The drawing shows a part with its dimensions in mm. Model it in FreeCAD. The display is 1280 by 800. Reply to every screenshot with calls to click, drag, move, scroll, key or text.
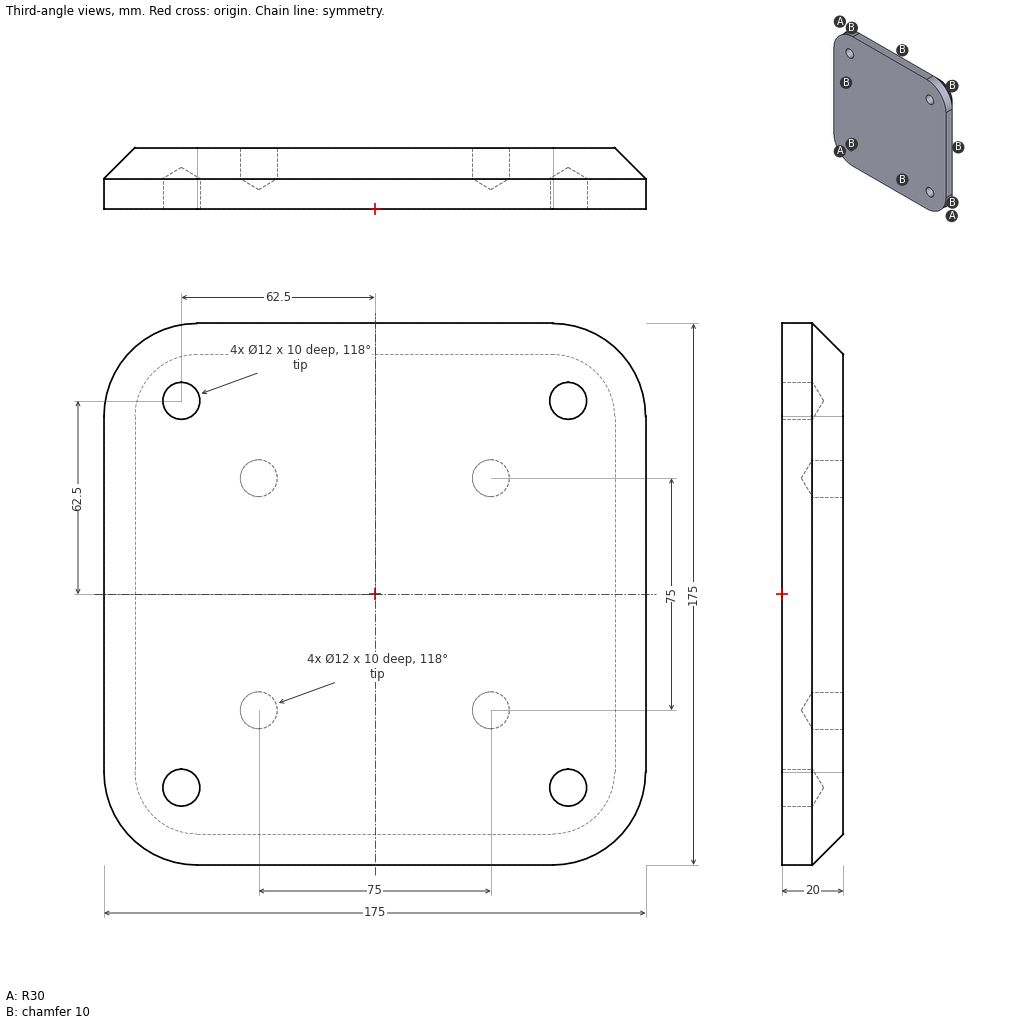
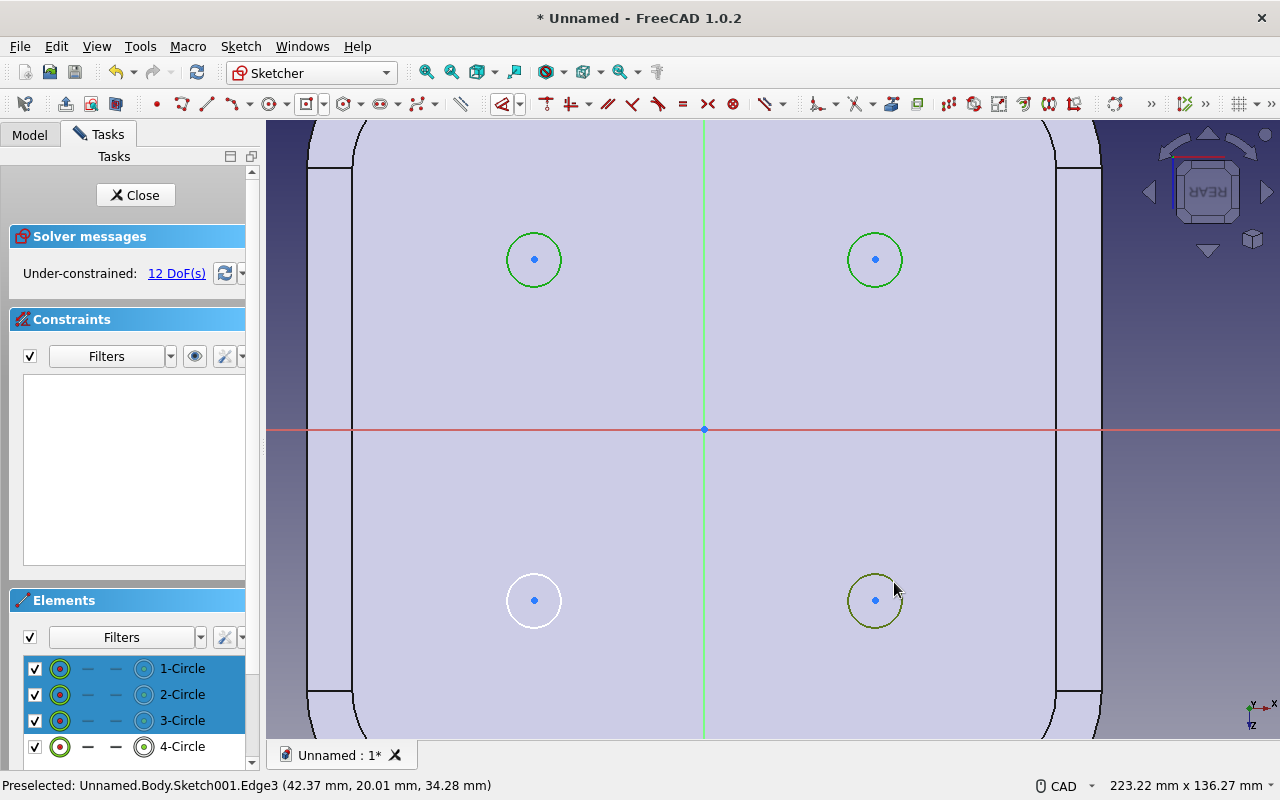
click(553, 582)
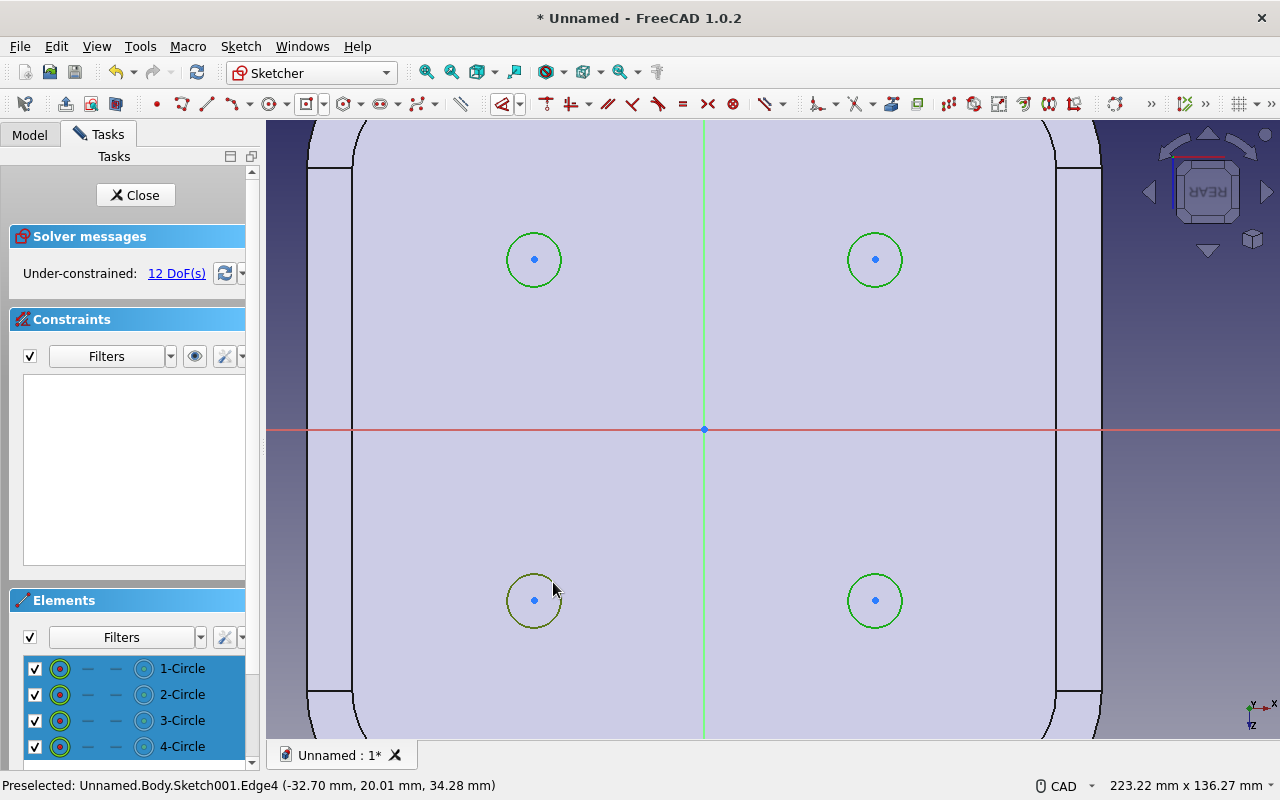
click(683, 104)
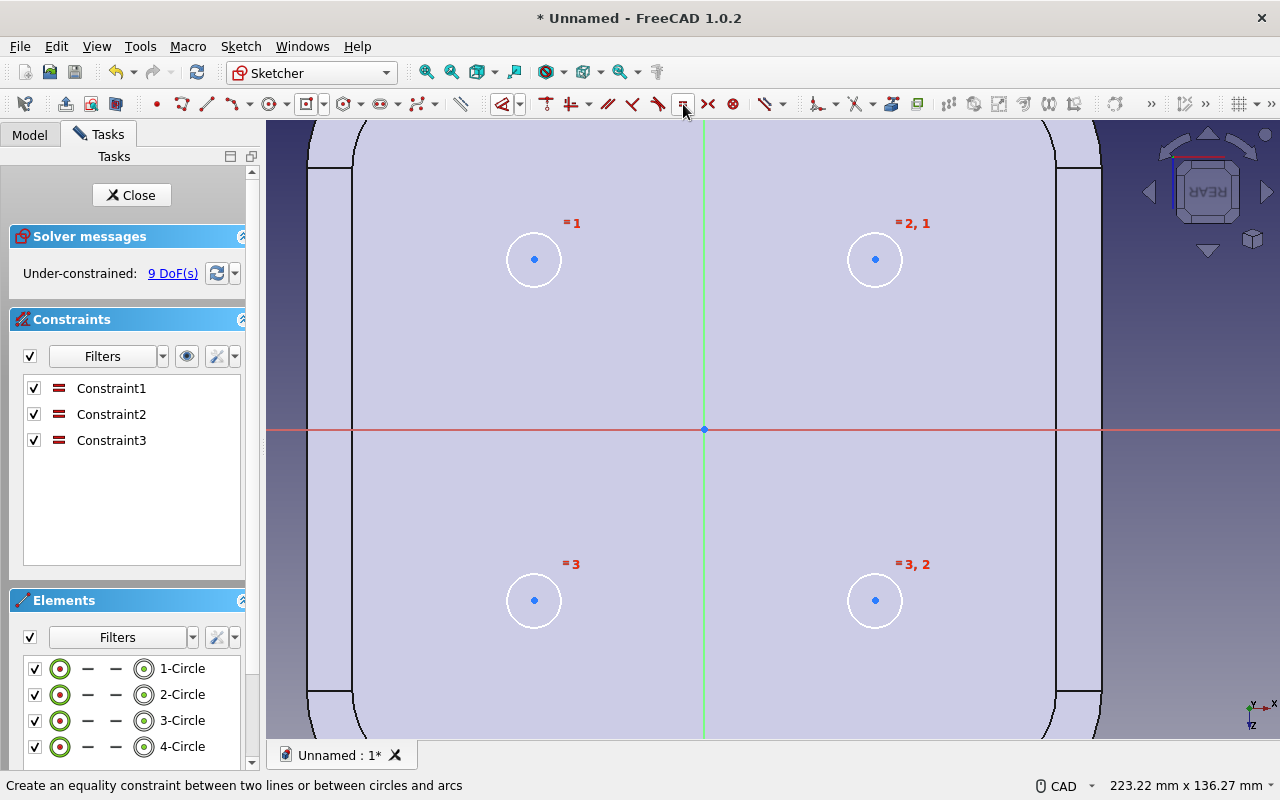
click(534, 260)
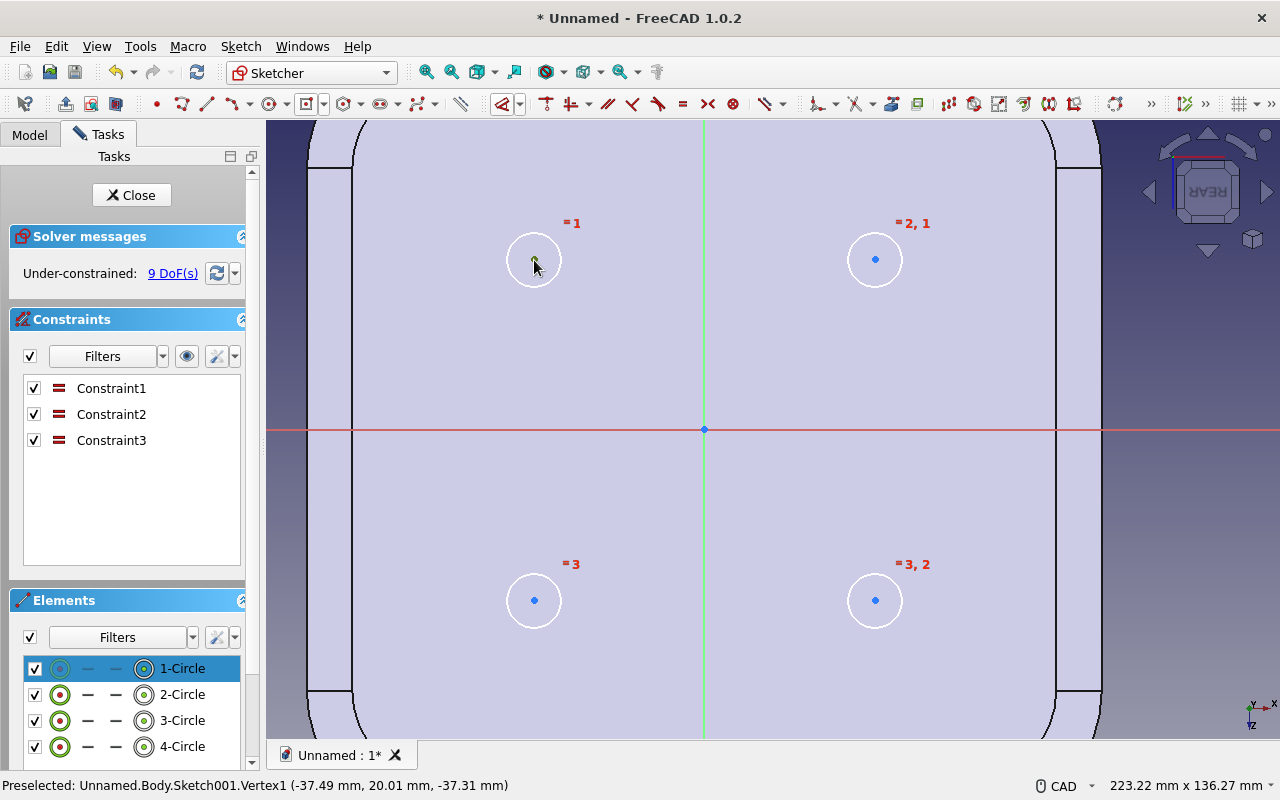
click(875, 260)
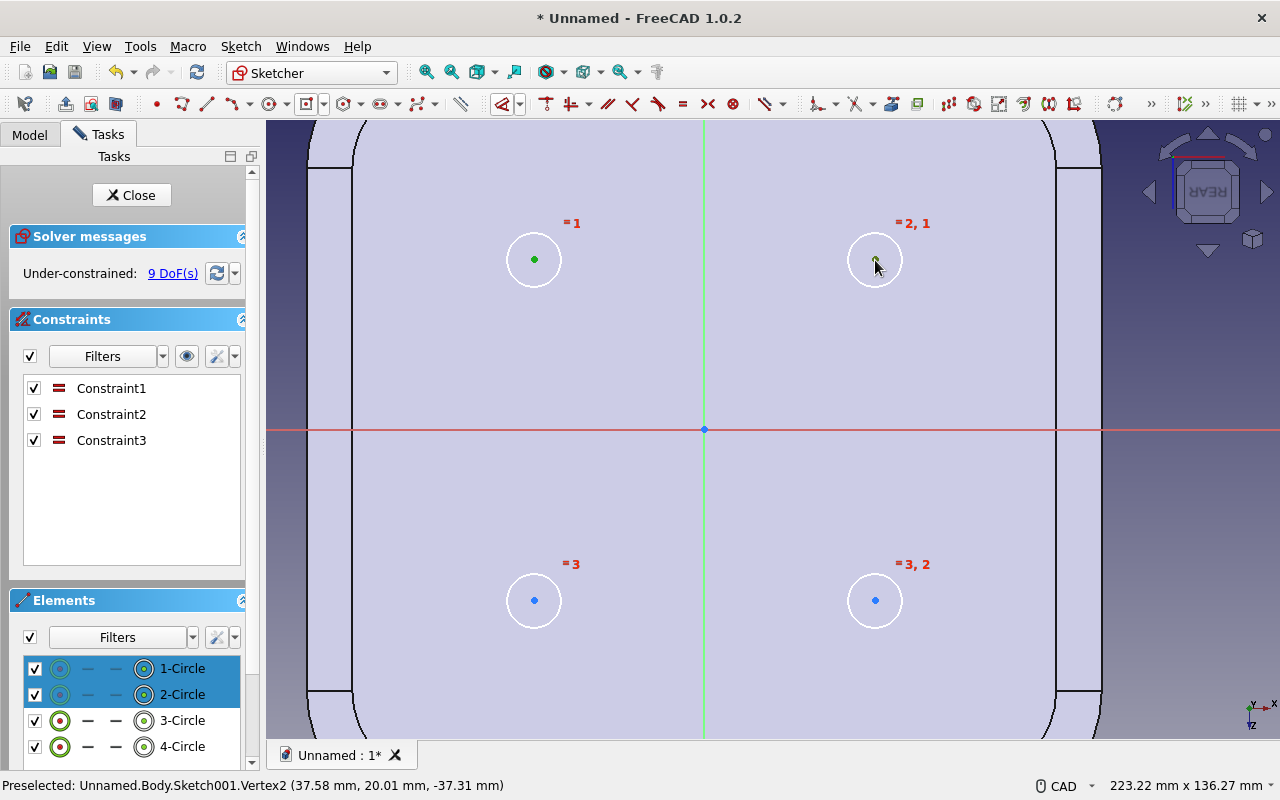
click(704, 671)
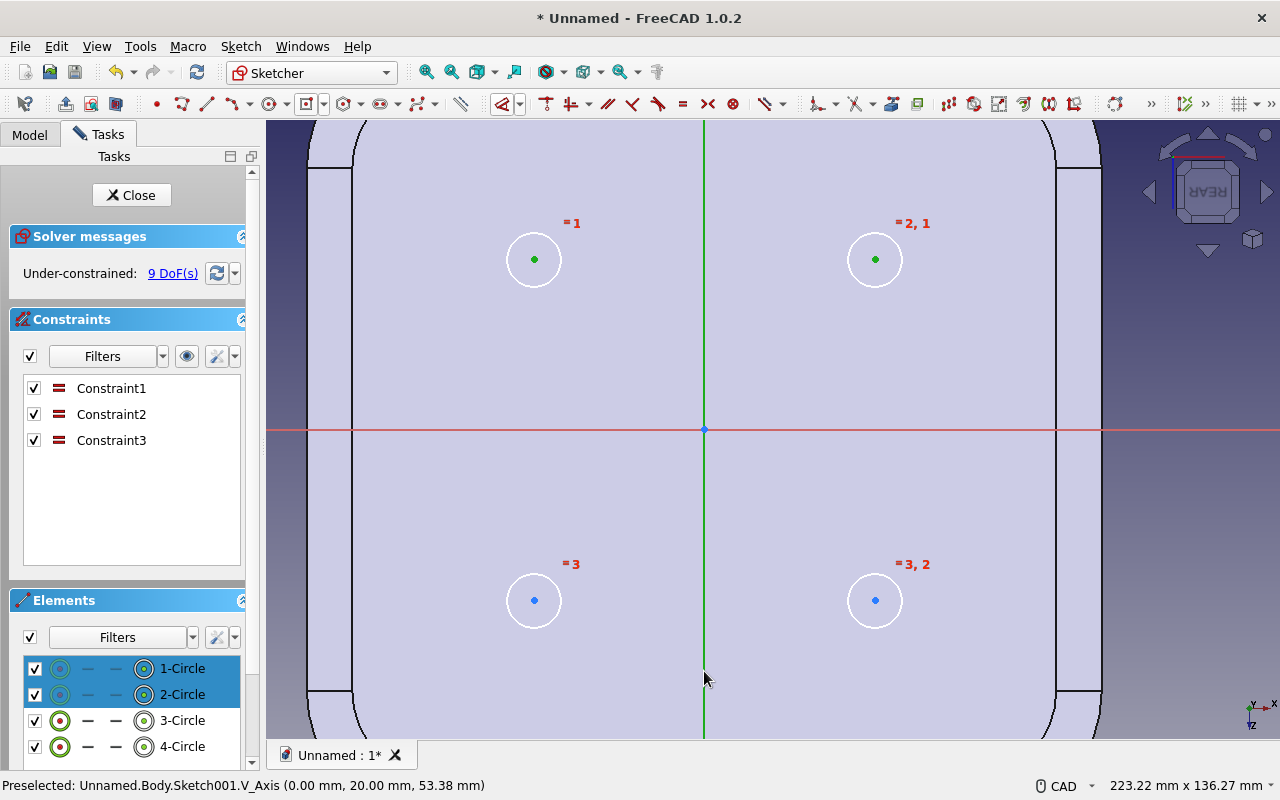
click(708, 104)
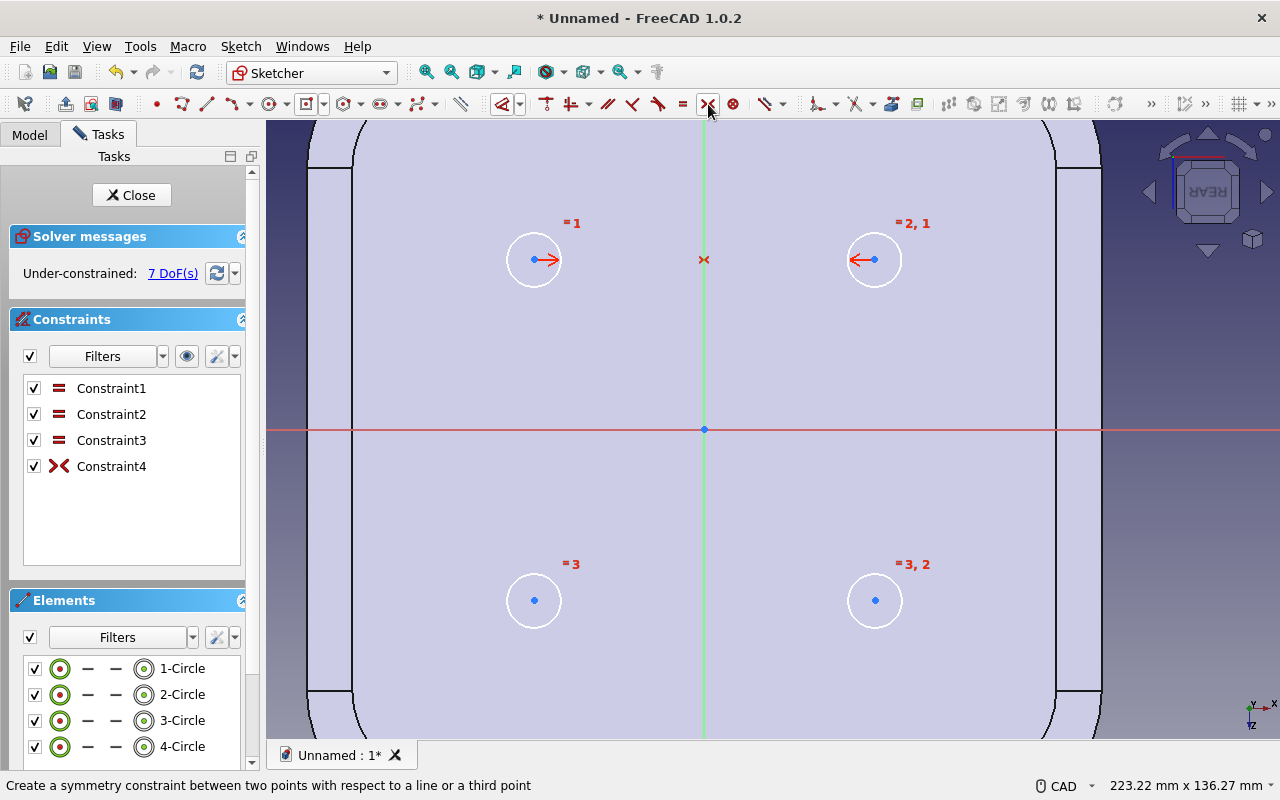
click(875, 260)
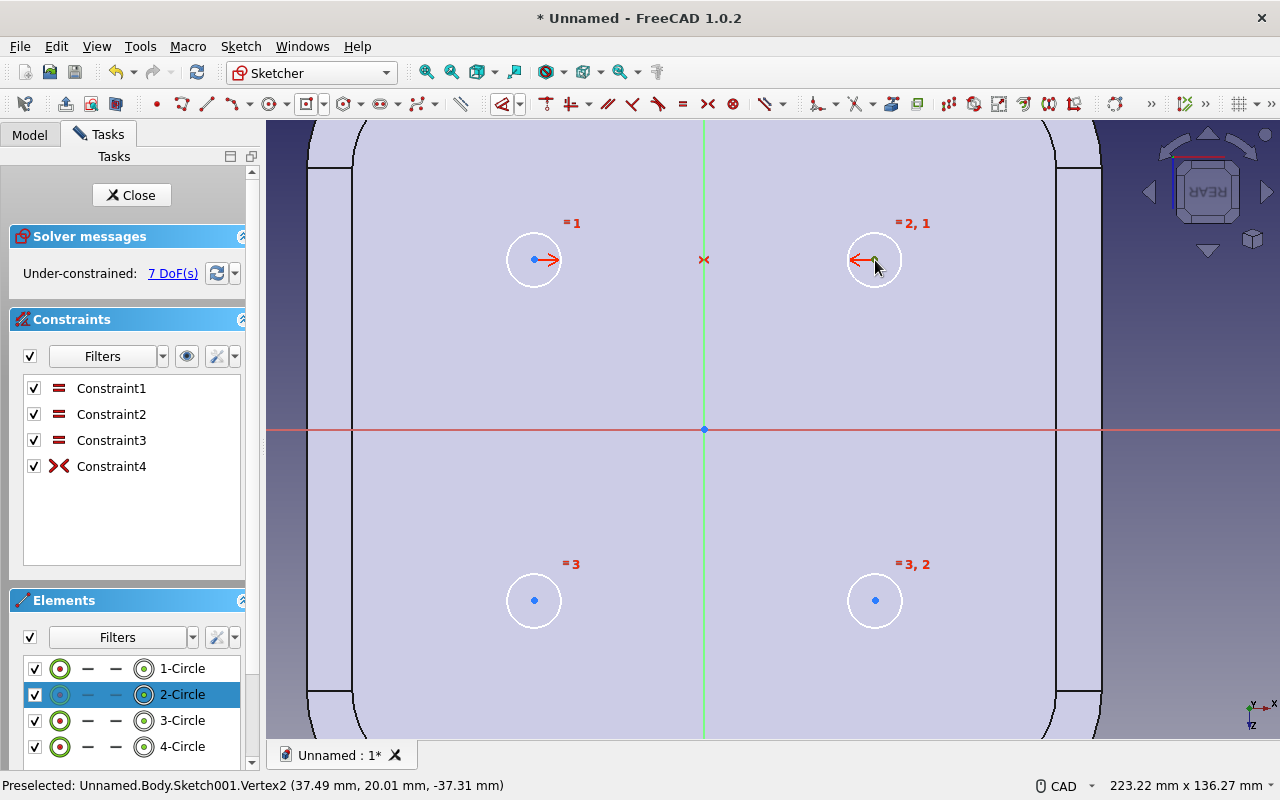
click(875, 601)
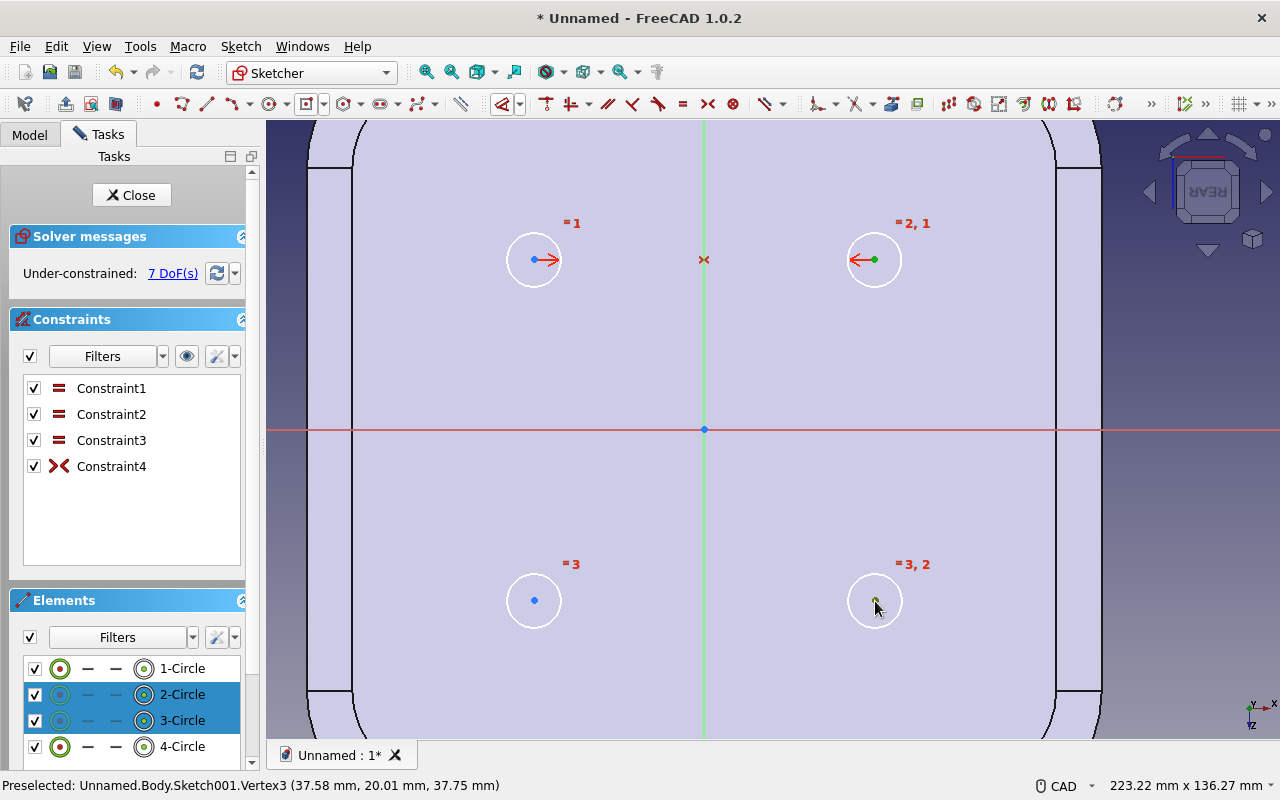
click(353, 429)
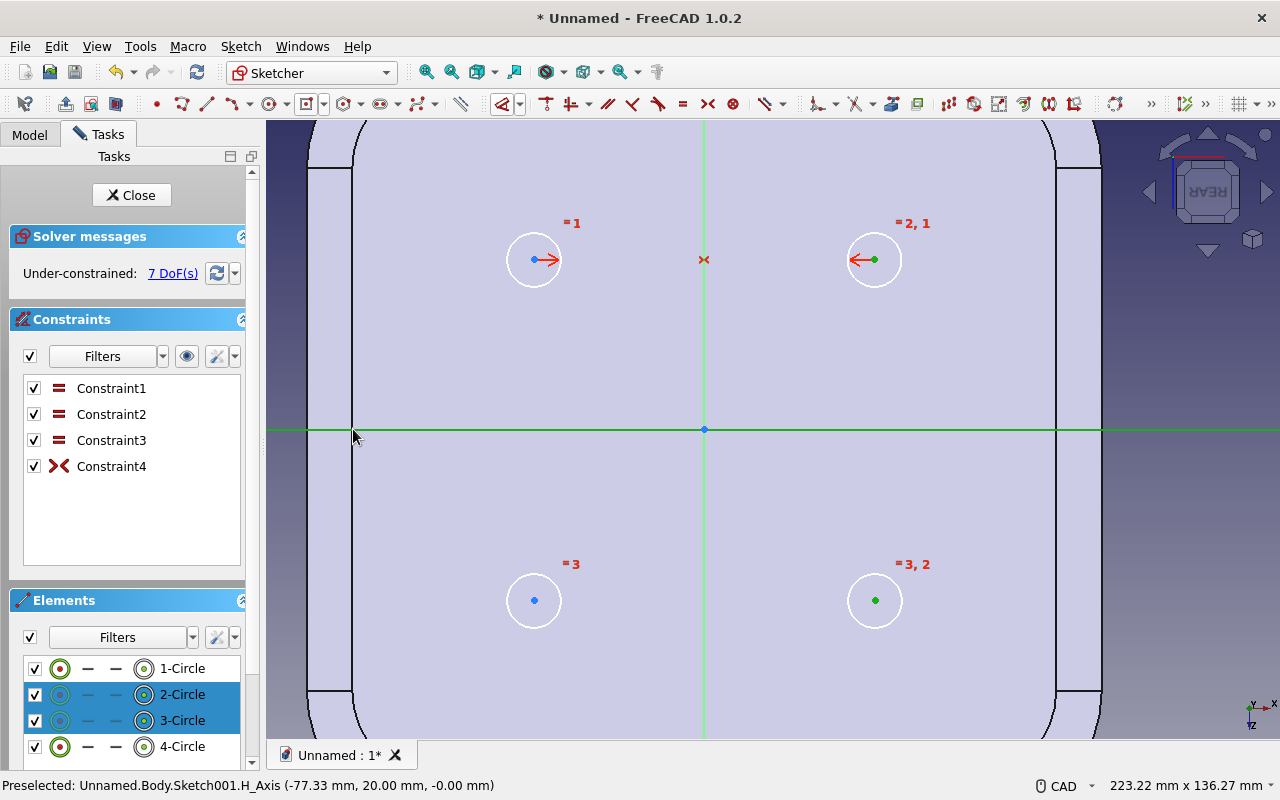
click(708, 104)